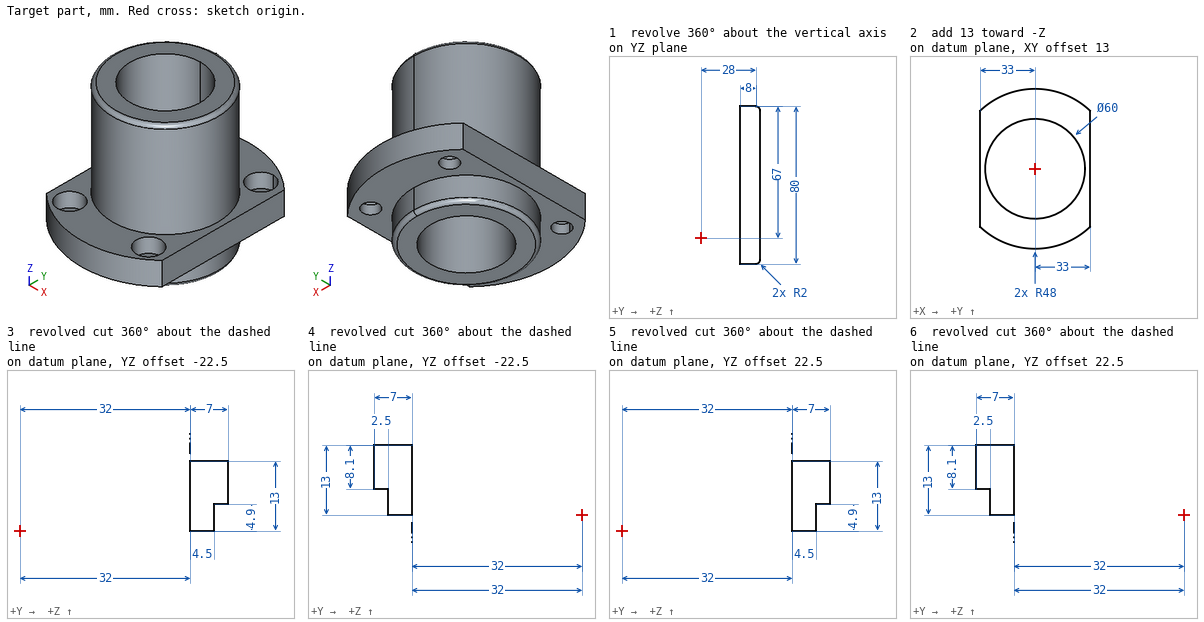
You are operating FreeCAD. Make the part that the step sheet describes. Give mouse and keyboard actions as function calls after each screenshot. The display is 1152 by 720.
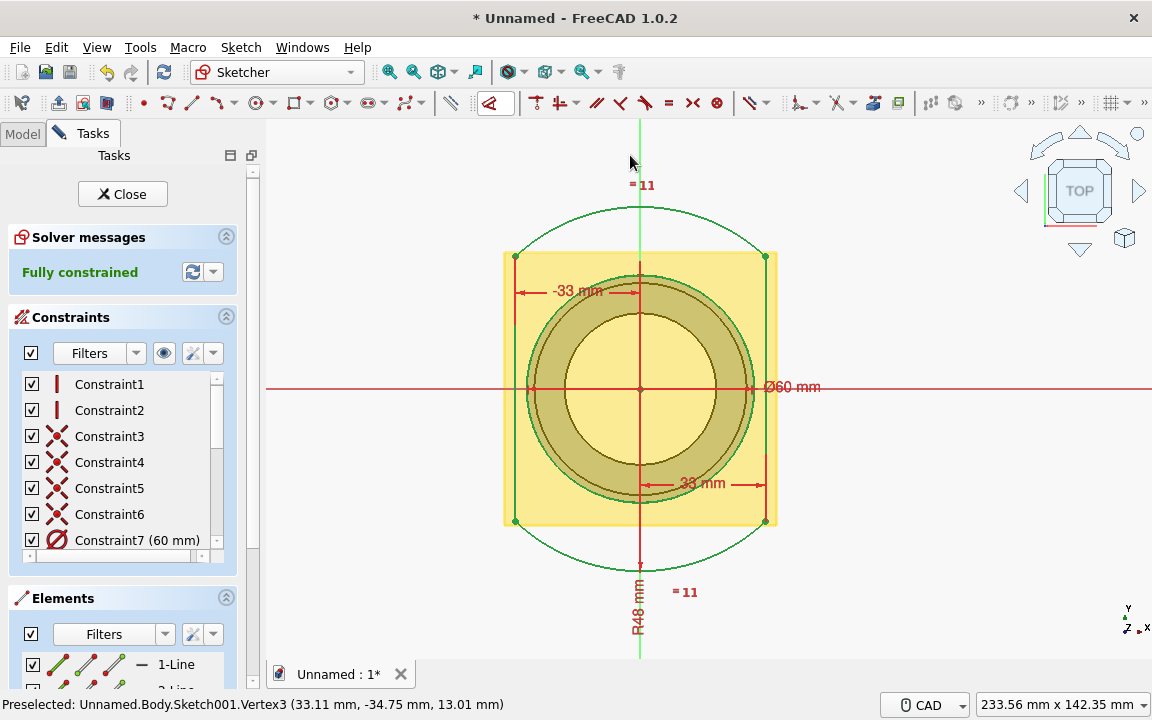
click(123, 194)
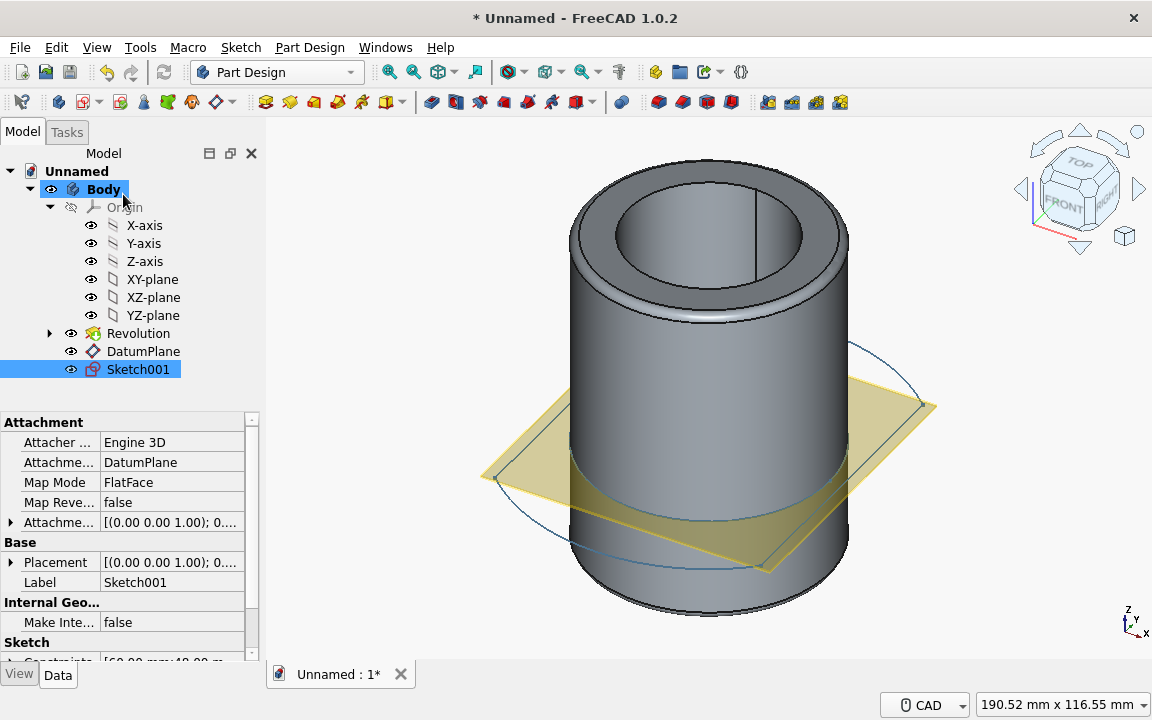
click(266, 102)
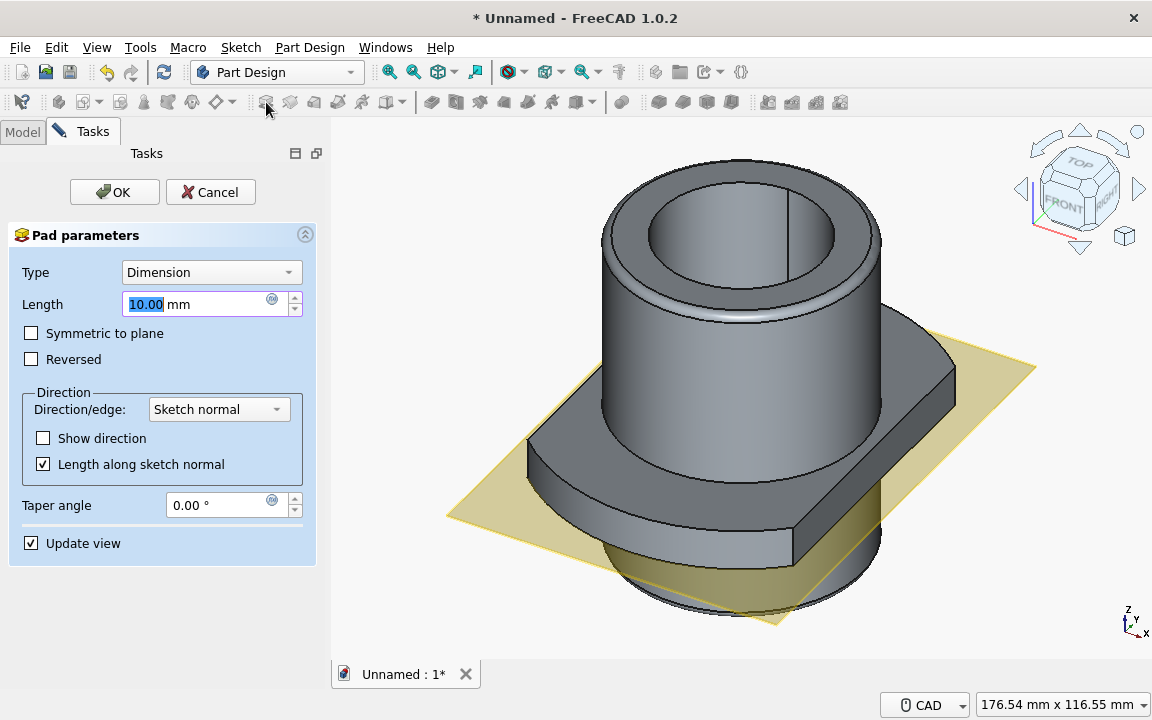
text(13)
key(Tab)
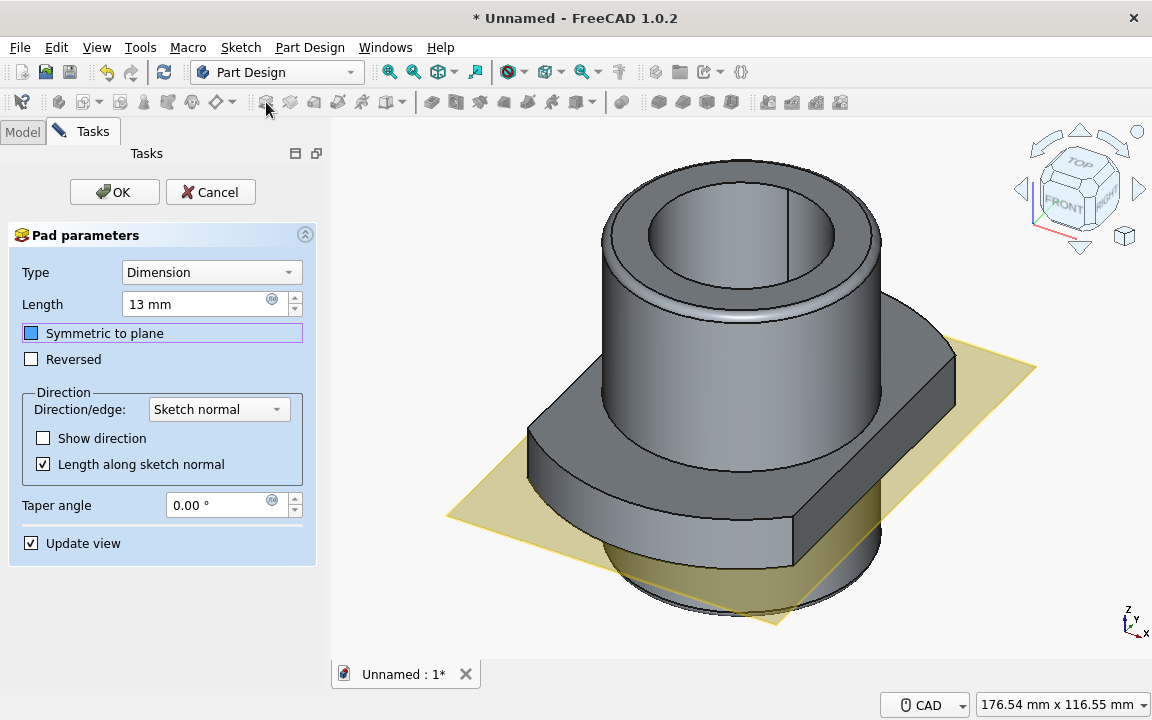
click(30, 359)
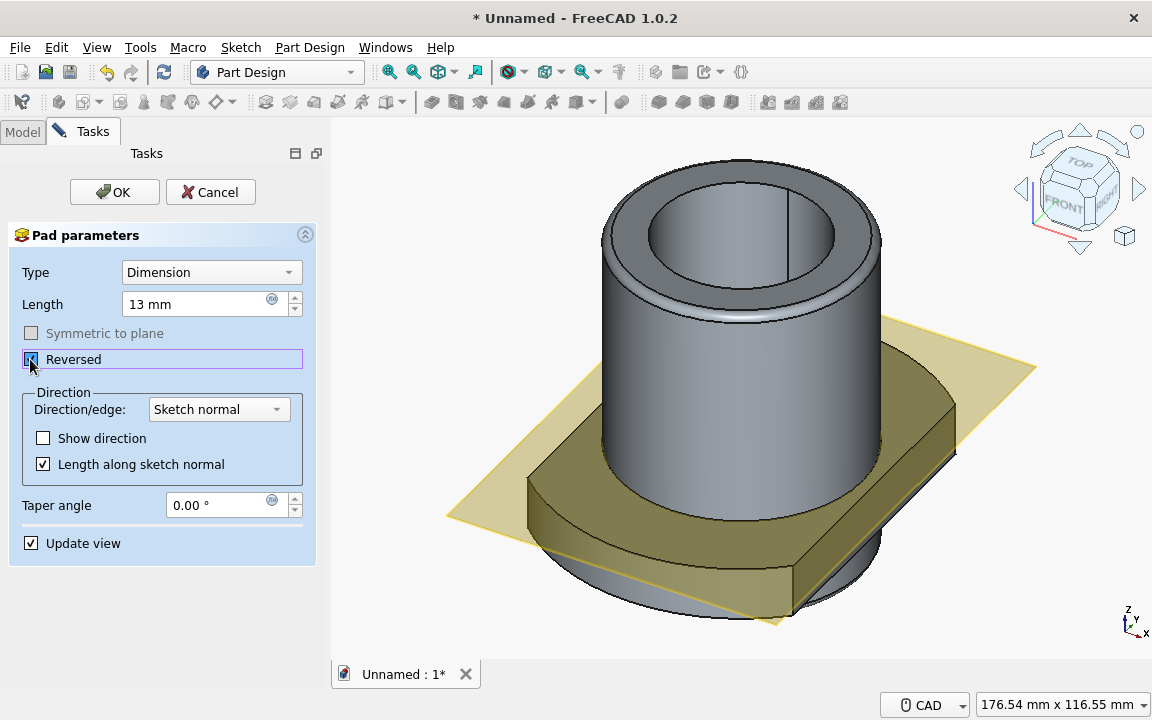
click(115, 192)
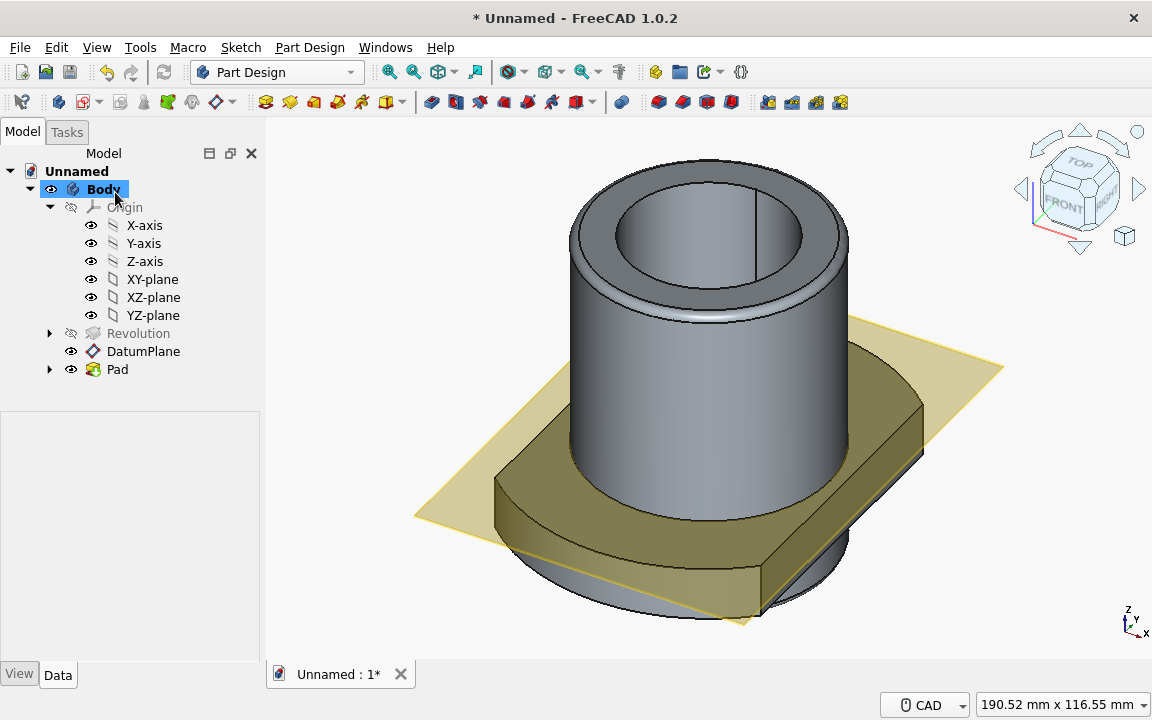
click(116, 351)
key(space)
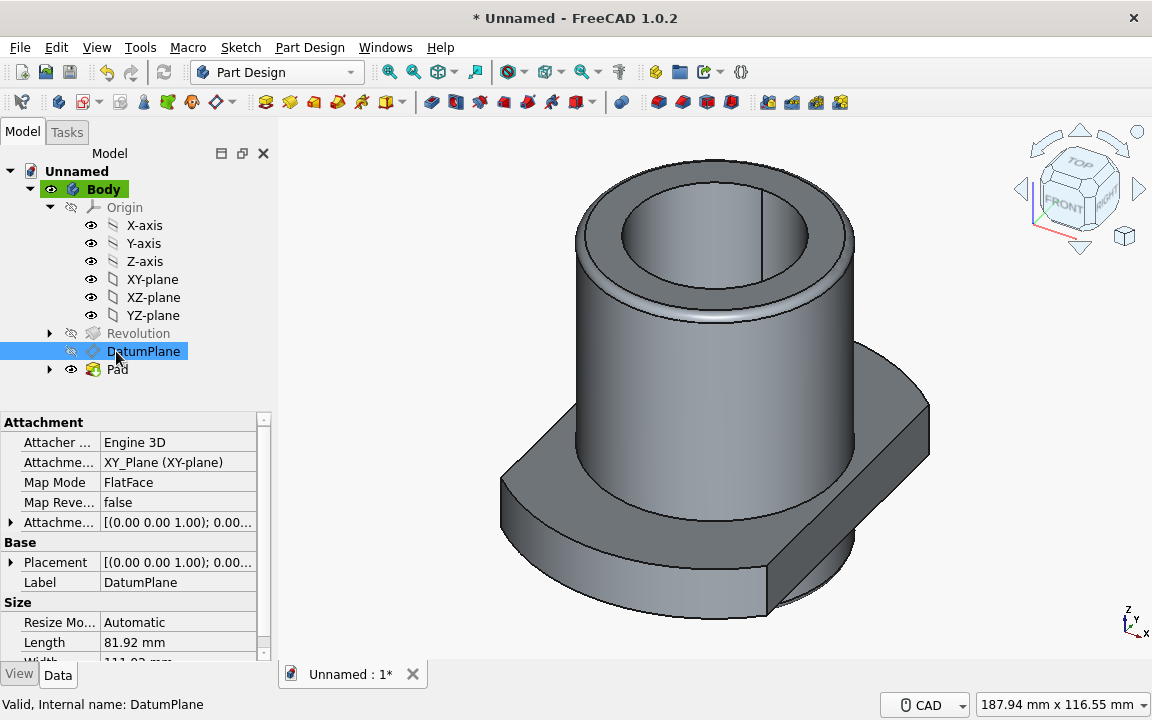
click(390, 72)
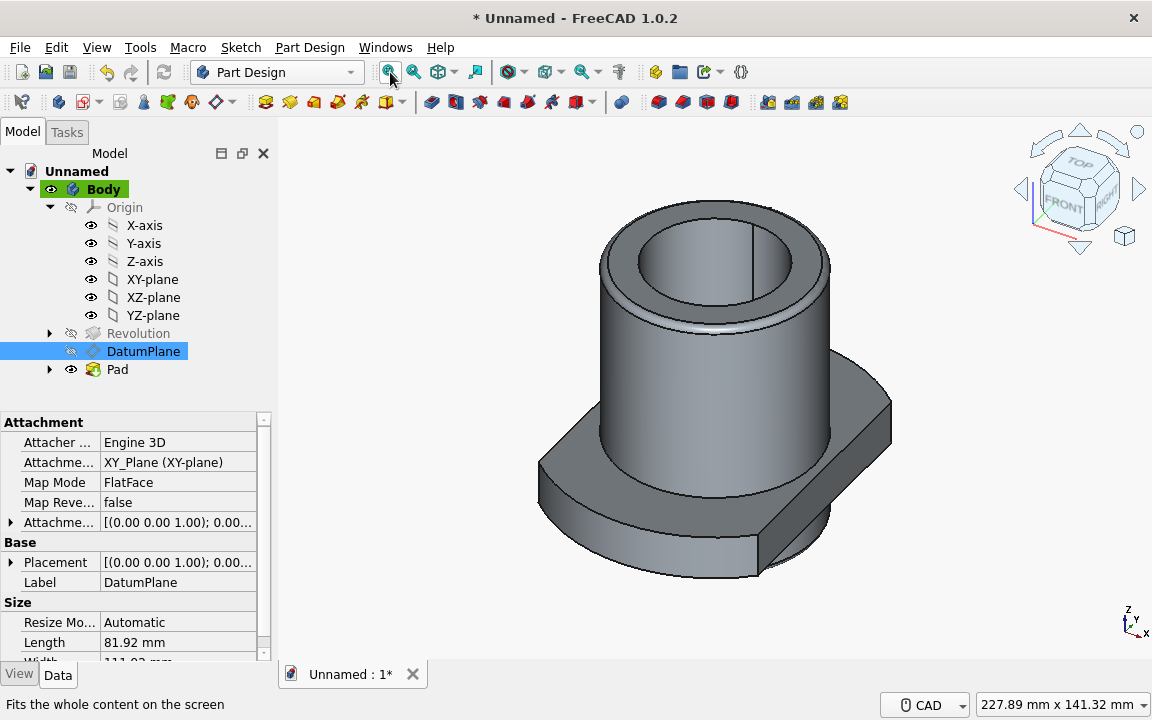
click(136, 315)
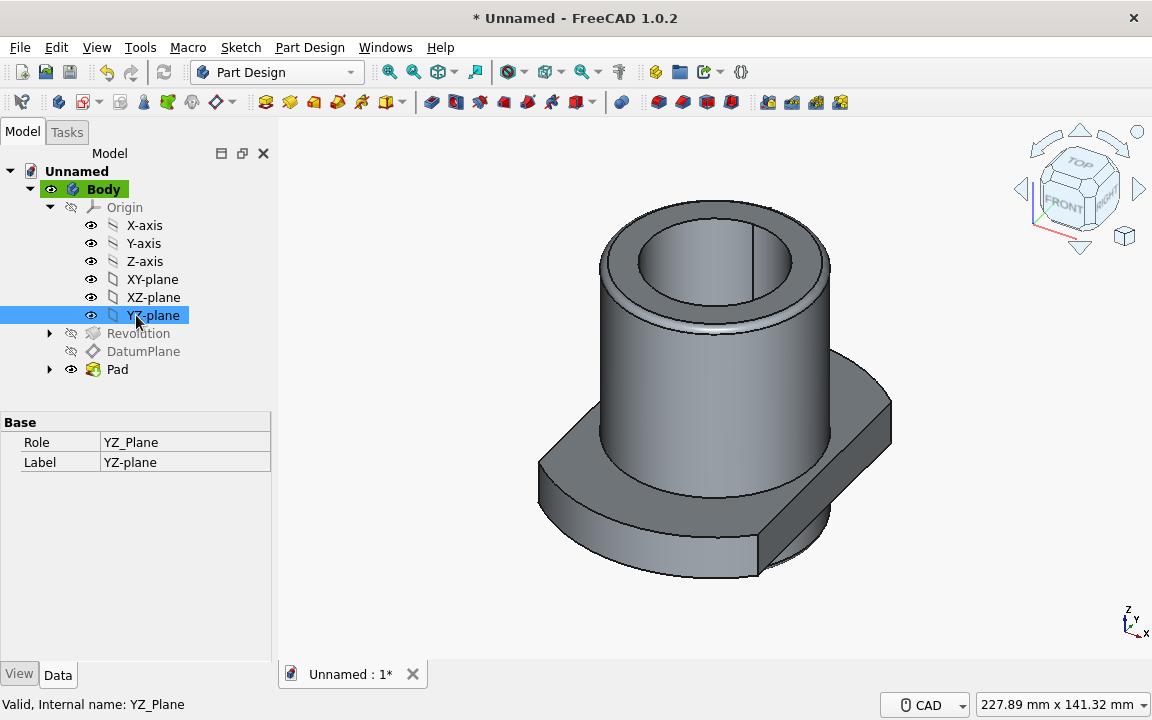
click(216, 102)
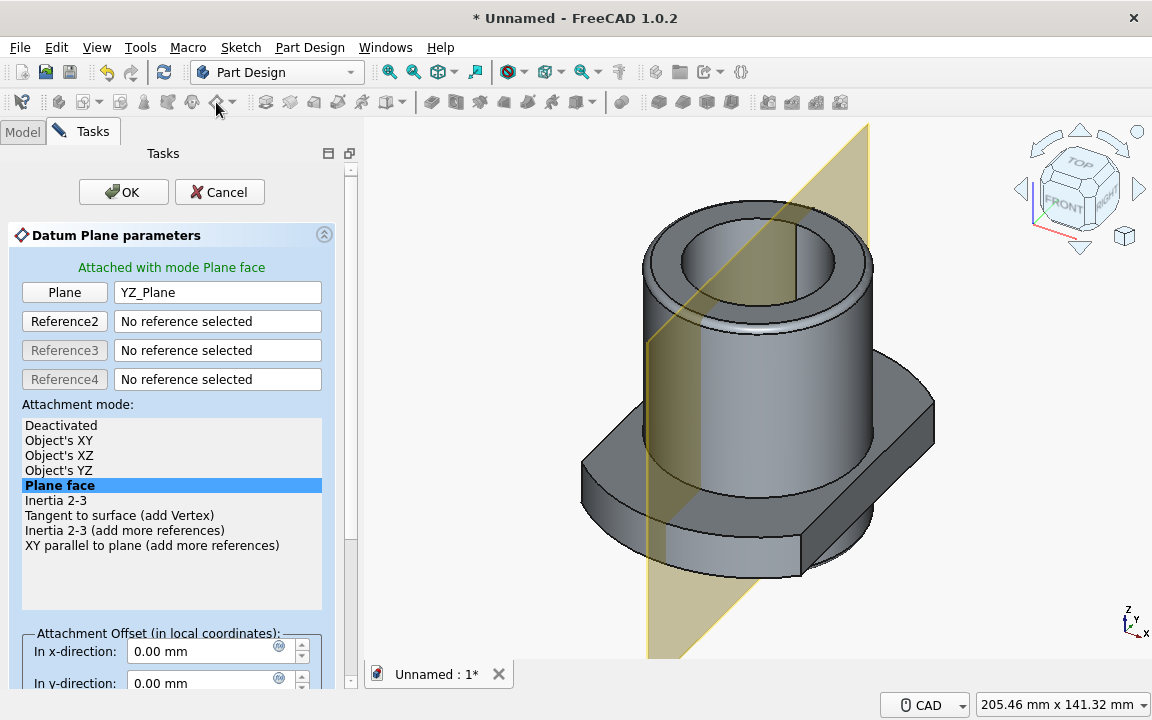
scroll(351, 426, down, 2)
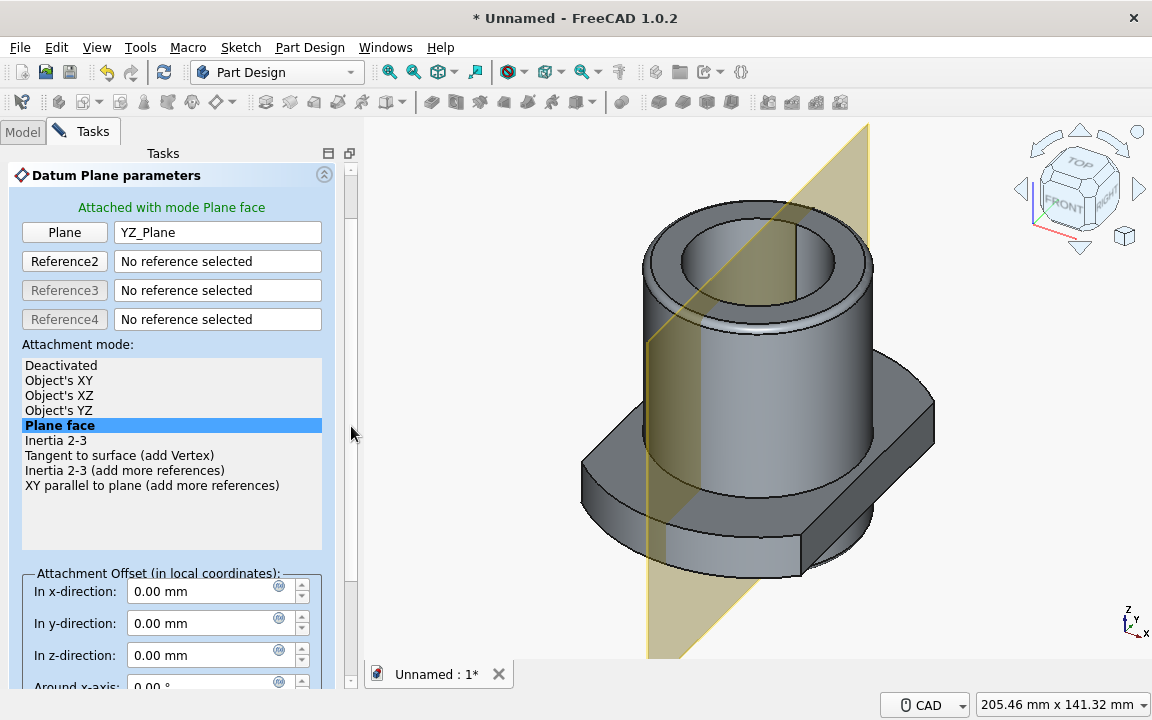
triple_click(210, 595)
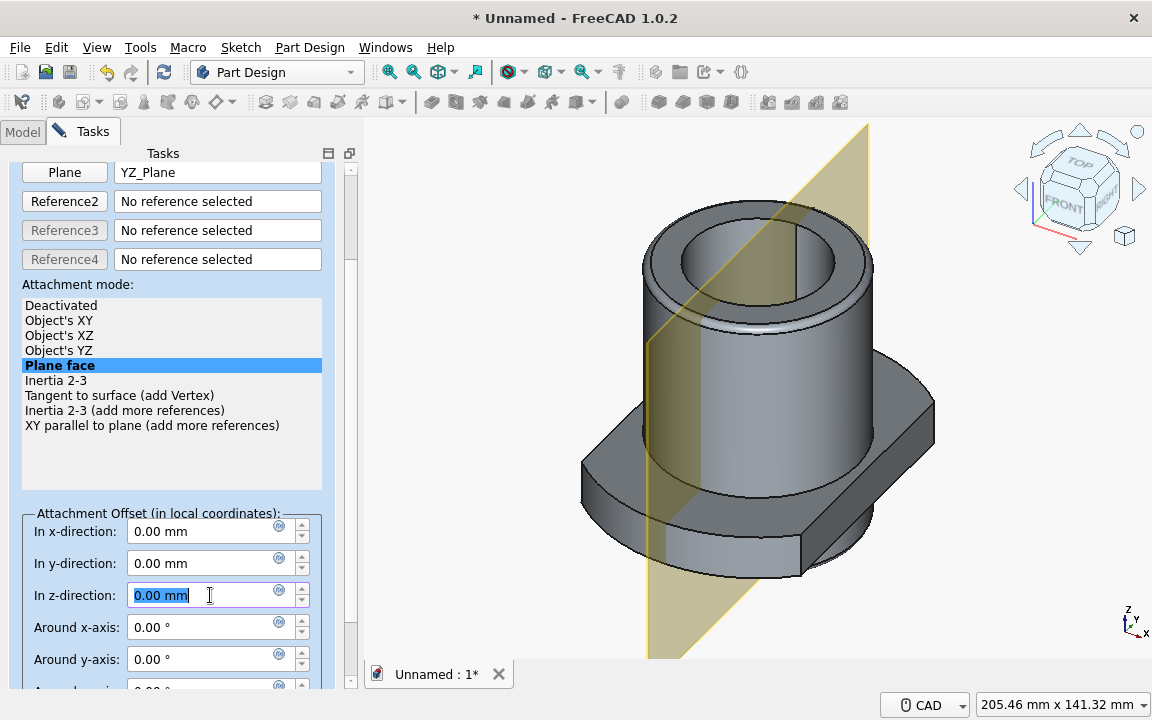
text(-22.5)
key(Tab)